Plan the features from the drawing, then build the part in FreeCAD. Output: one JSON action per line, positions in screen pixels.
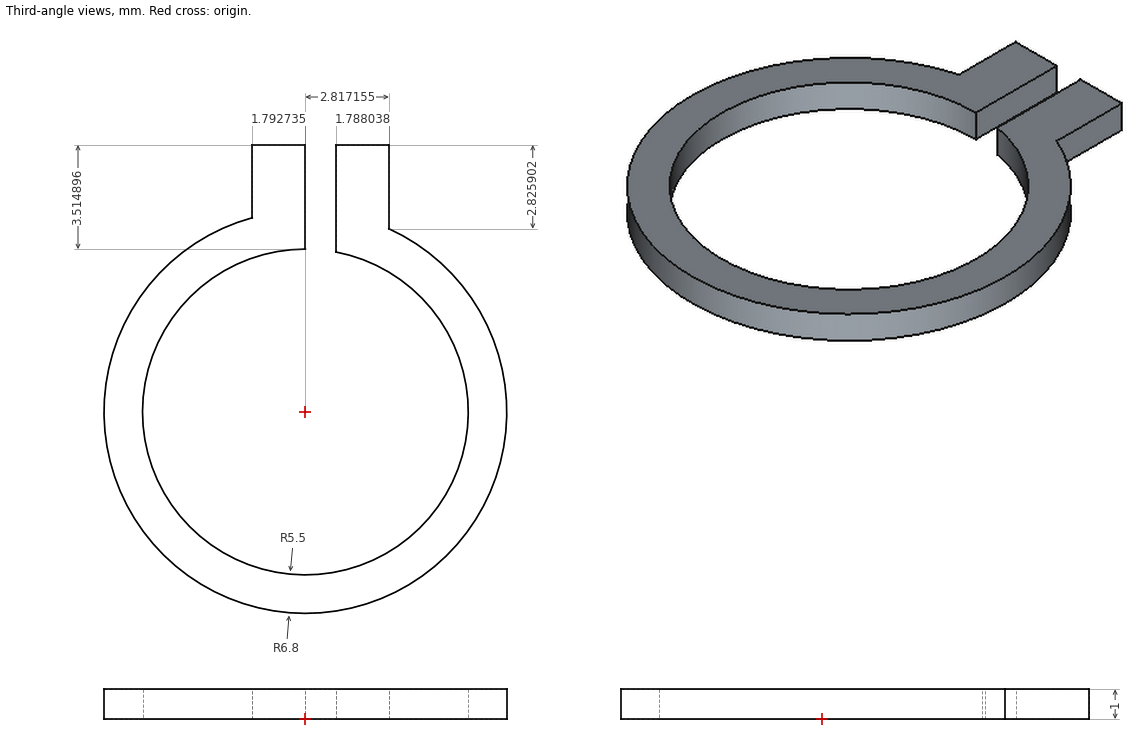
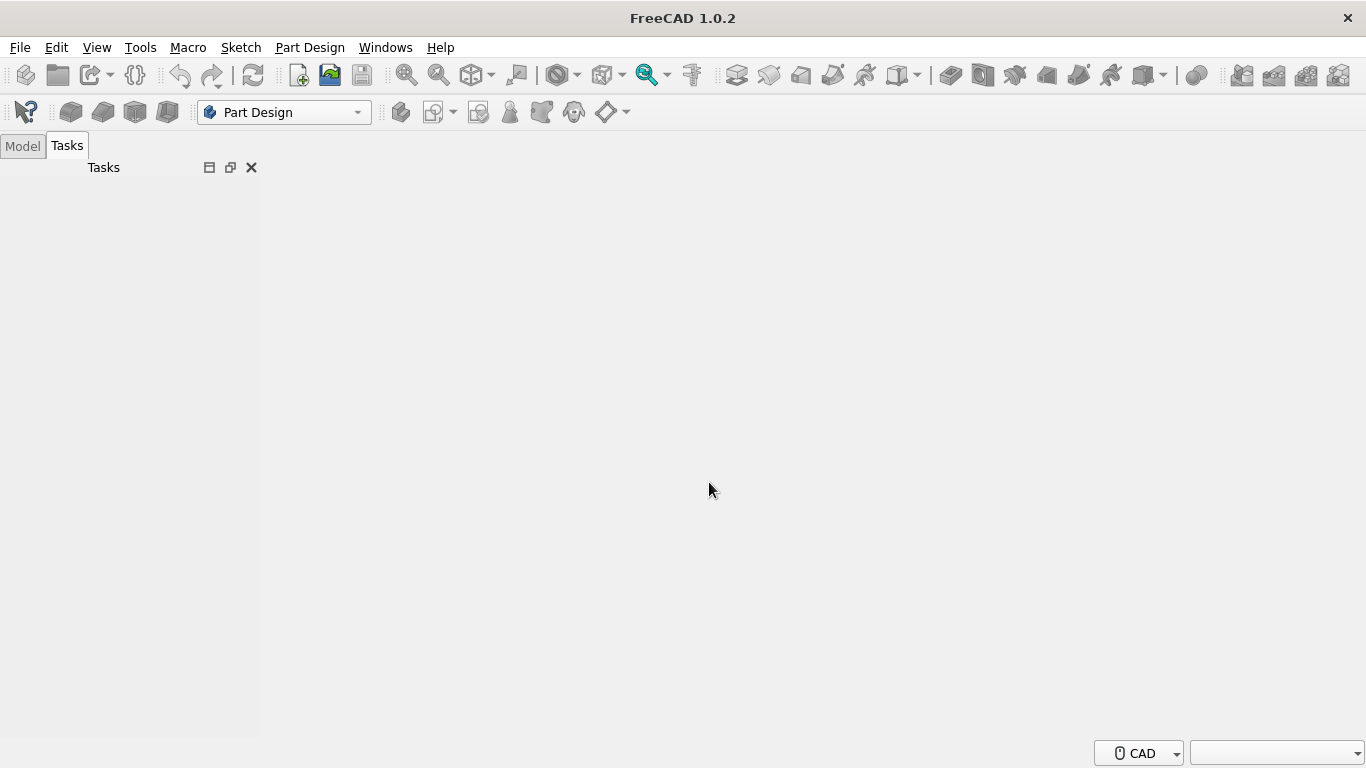
{"action": "left_click", "coordinate": [298, 76]}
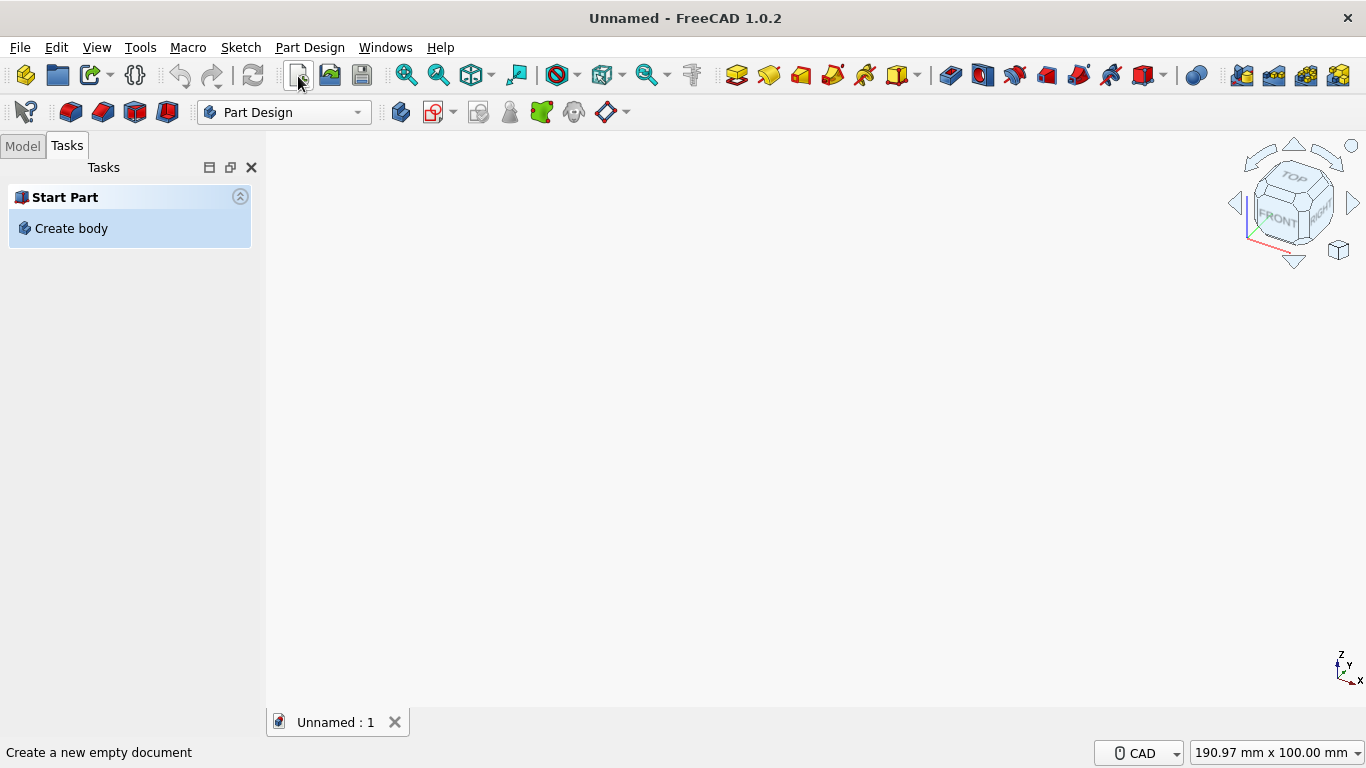
{"action": "left_click", "coordinate": [434, 112]}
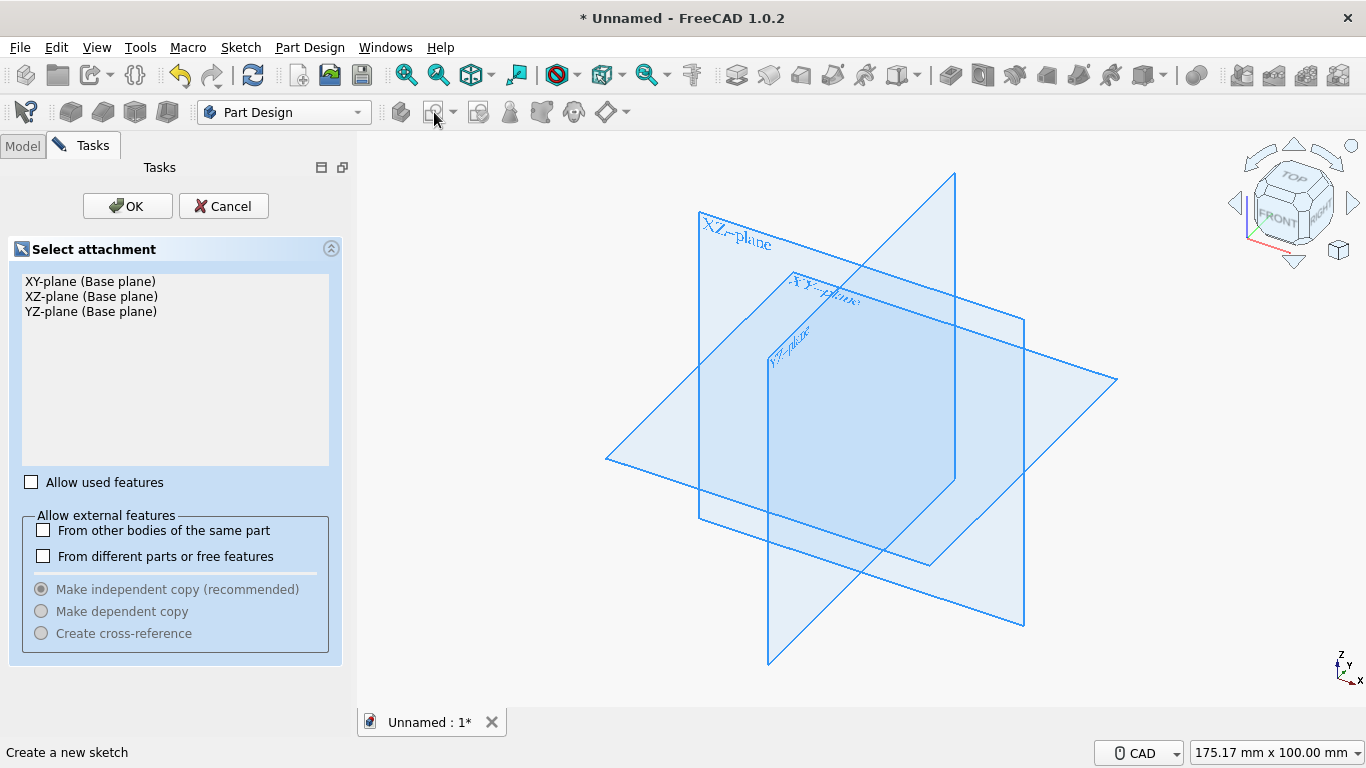
{"action": "left_click", "coordinate": [82, 282]}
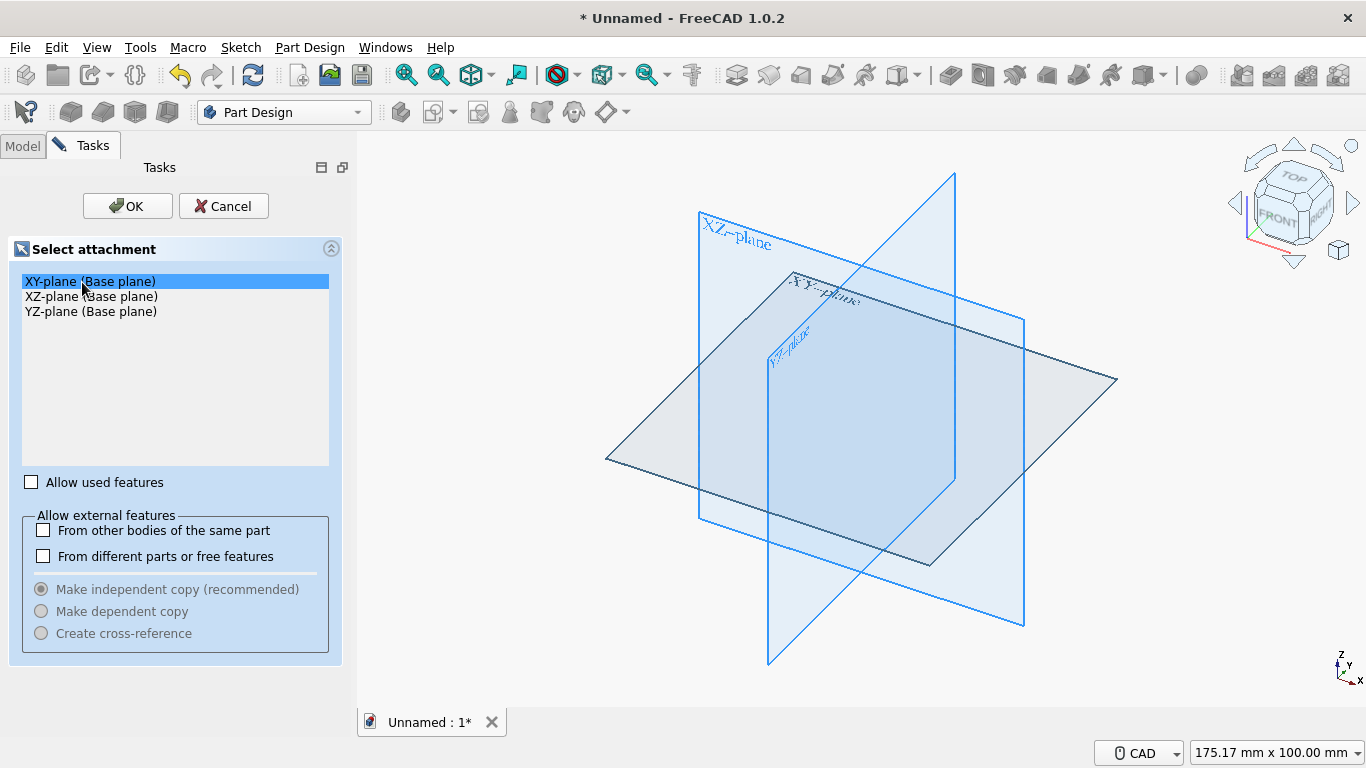
{"action": "left_click", "coordinate": [128, 206]}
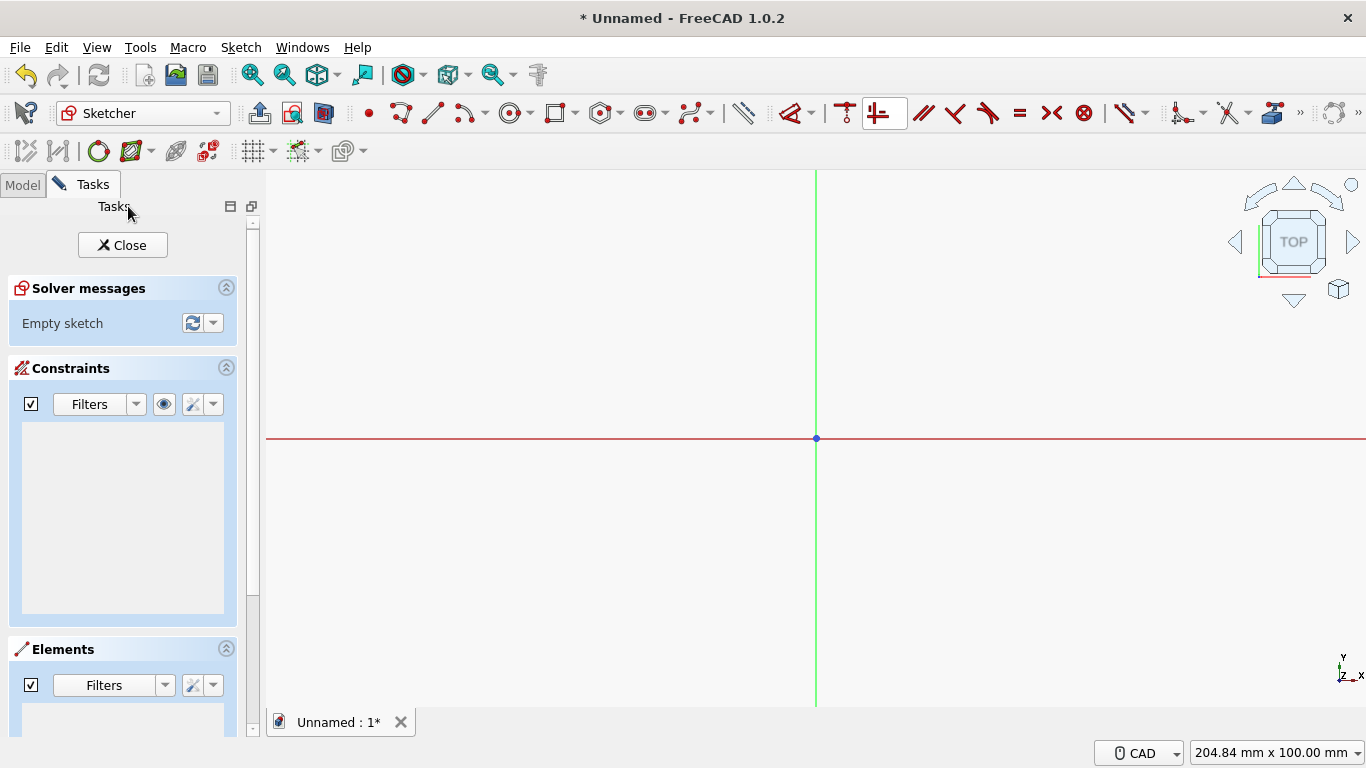
{"action": "scroll", "coordinate": [842, 431], "scroll_direction": "up", "scroll_amount": 7}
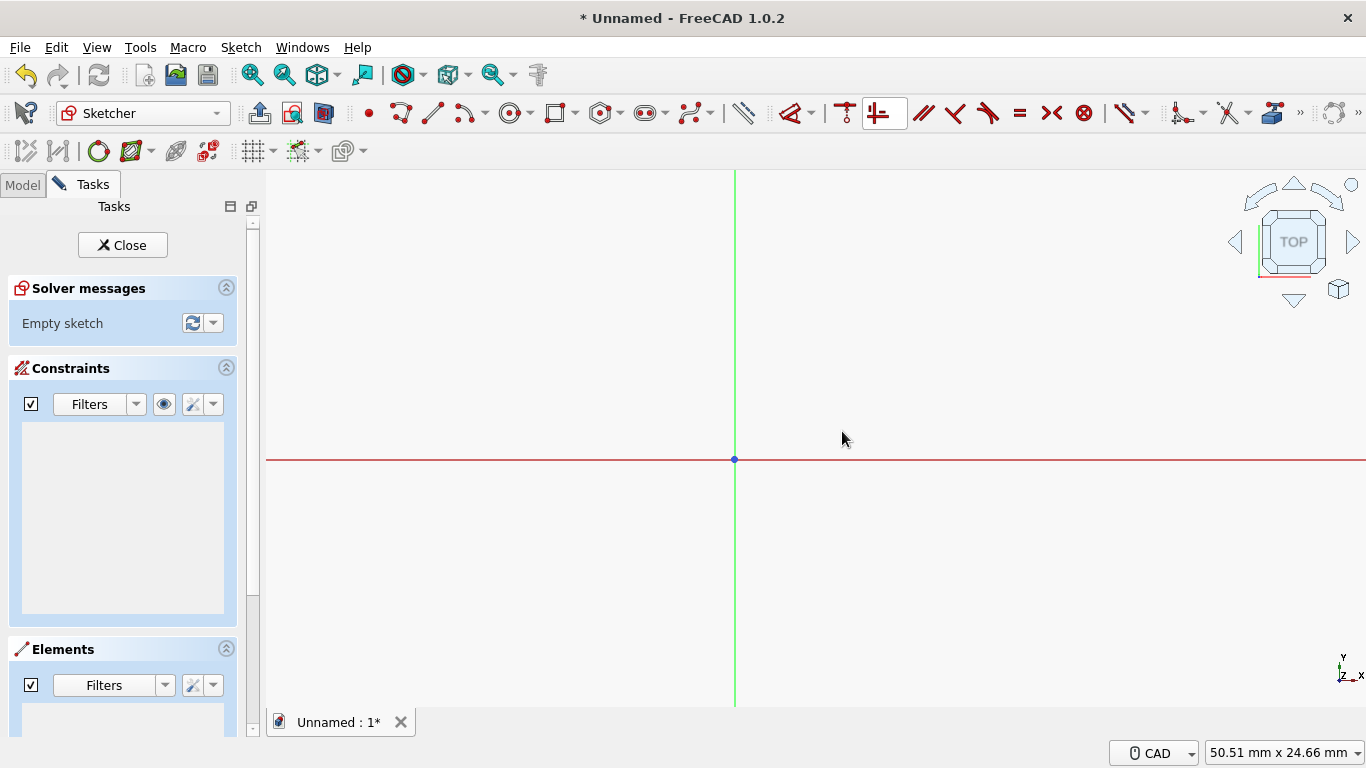
{"action": "left_click", "coordinate": [402, 114]}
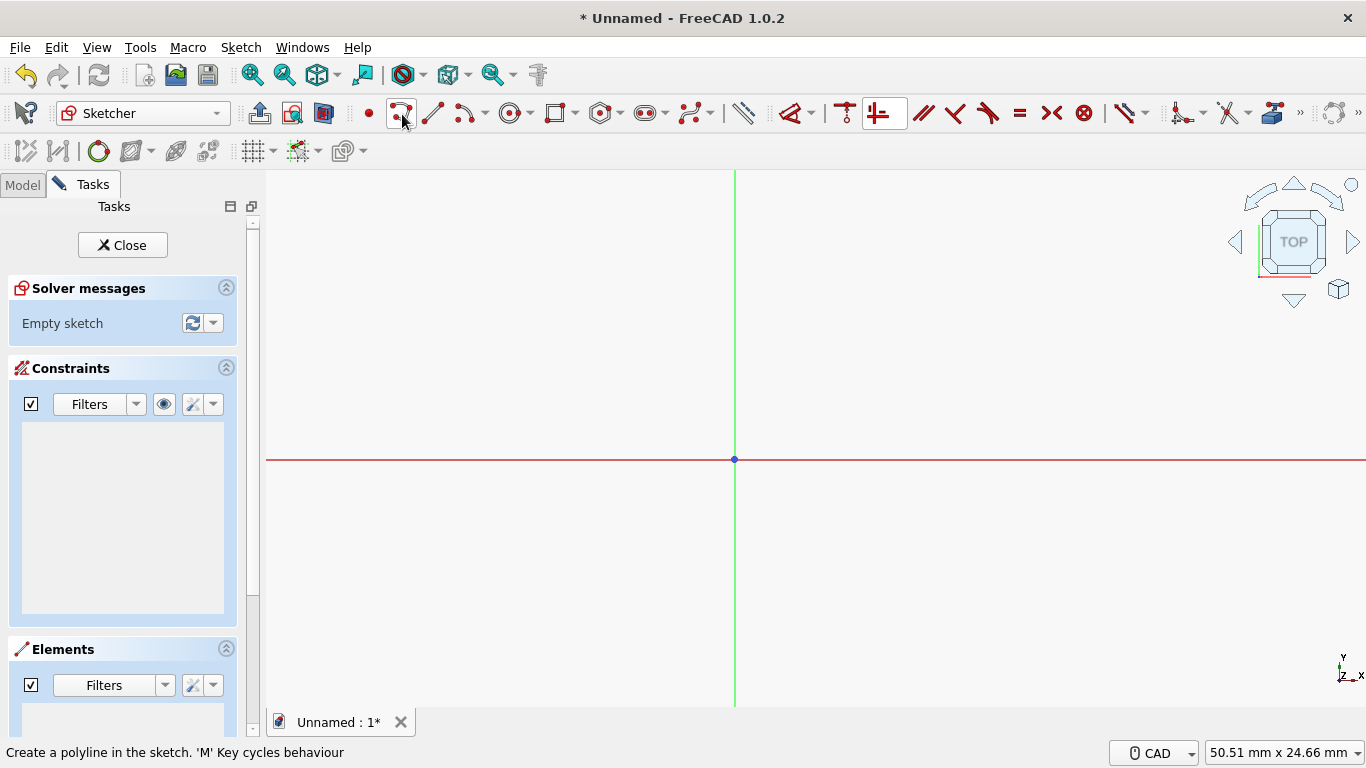
{"action": "left_click", "coordinate": [735, 340]}
{"action": "left_click", "coordinate": [744, 264]}
{"action": "left_click", "coordinate": [696, 264]}
{"action": "left_click", "coordinate": [696, 317]}
{"action": "right_click", "coordinate": [696, 317]}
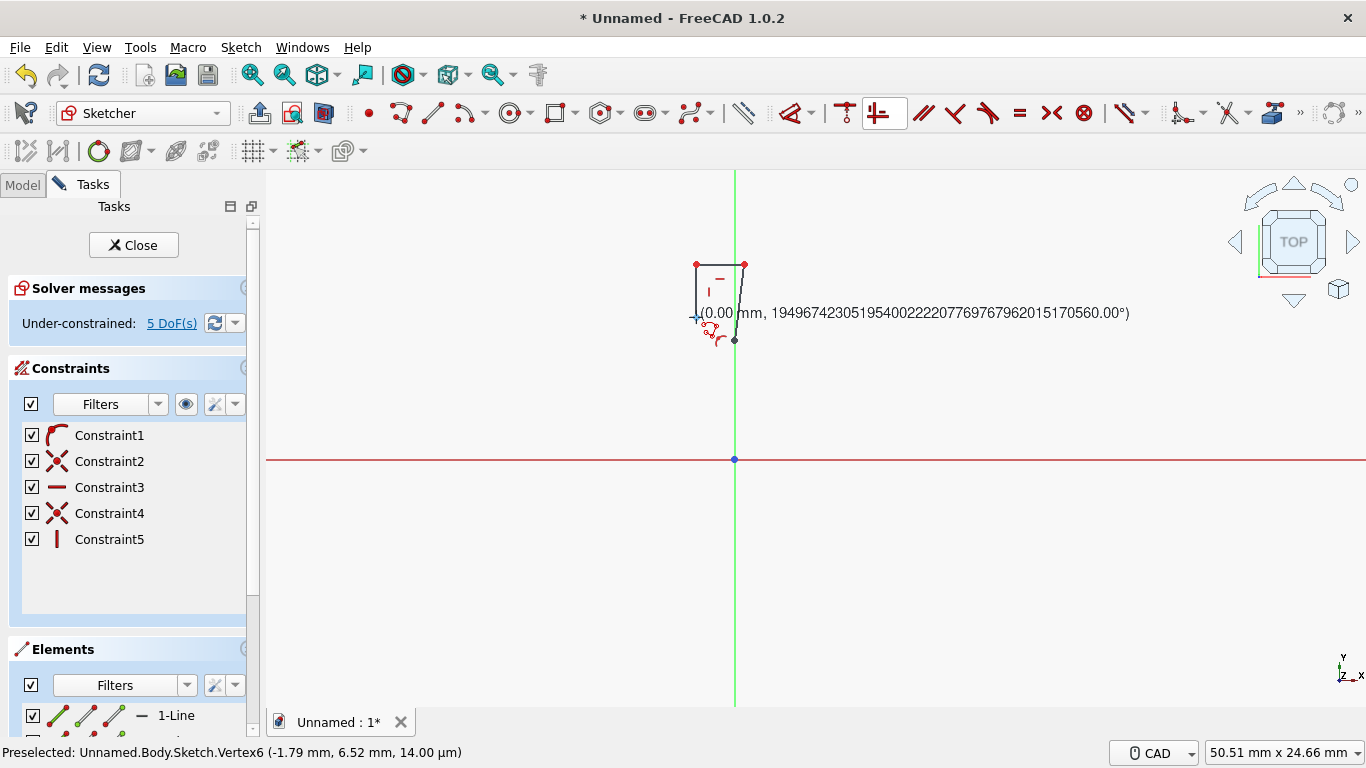
{"action": "left_click", "coordinate": [796, 325]}
{"action": "left_click", "coordinate": [796, 264]}
{"action": "left_click", "coordinate": [757, 264]}
{"action": "left_click", "coordinate": [757, 342]}
{"action": "right_click", "coordinate": [757, 342]}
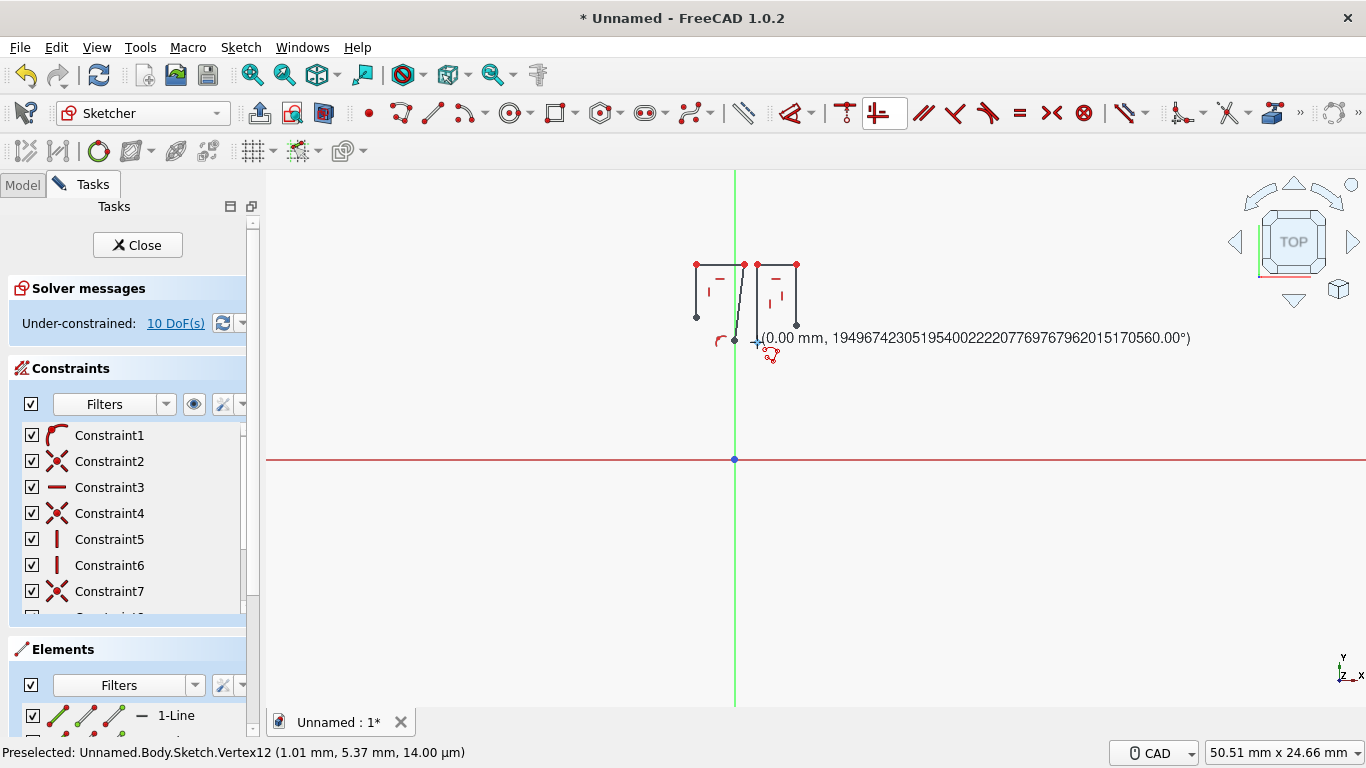
{"action": "left_click", "coordinate": [488, 114]}